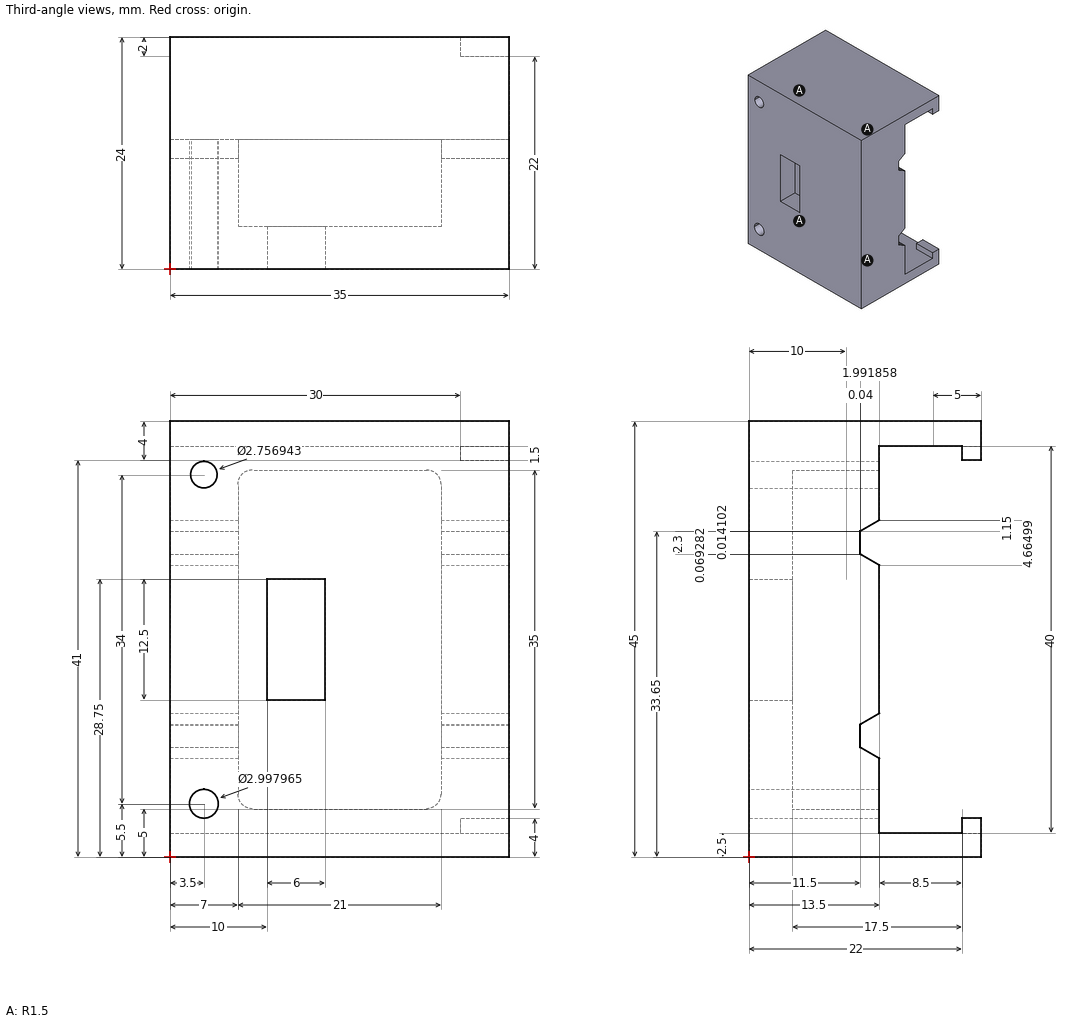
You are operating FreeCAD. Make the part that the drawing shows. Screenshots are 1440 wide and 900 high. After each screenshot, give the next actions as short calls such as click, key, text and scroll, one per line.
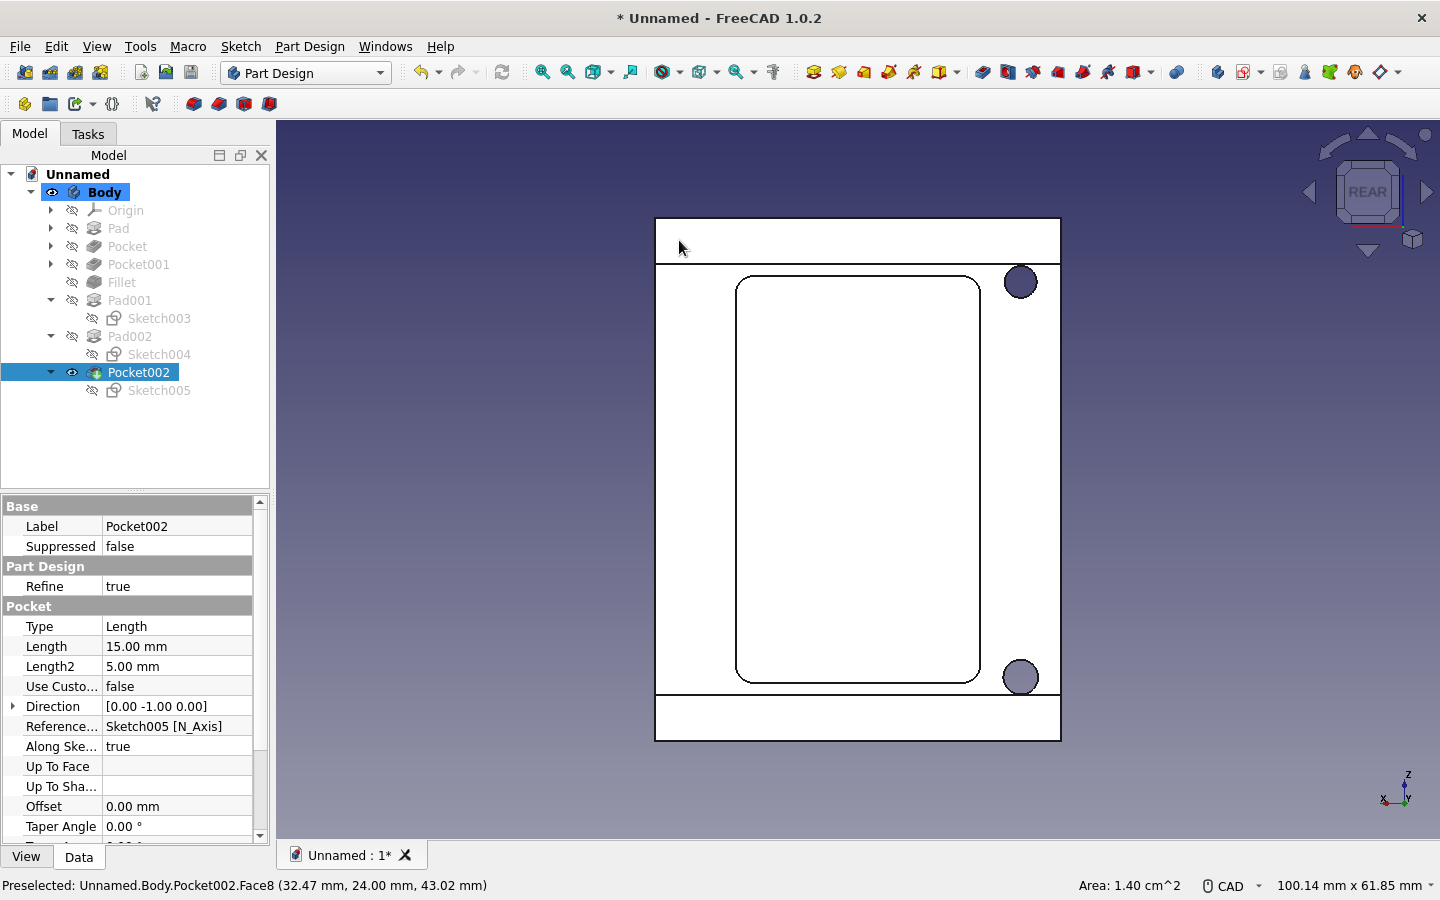
click(1242, 72)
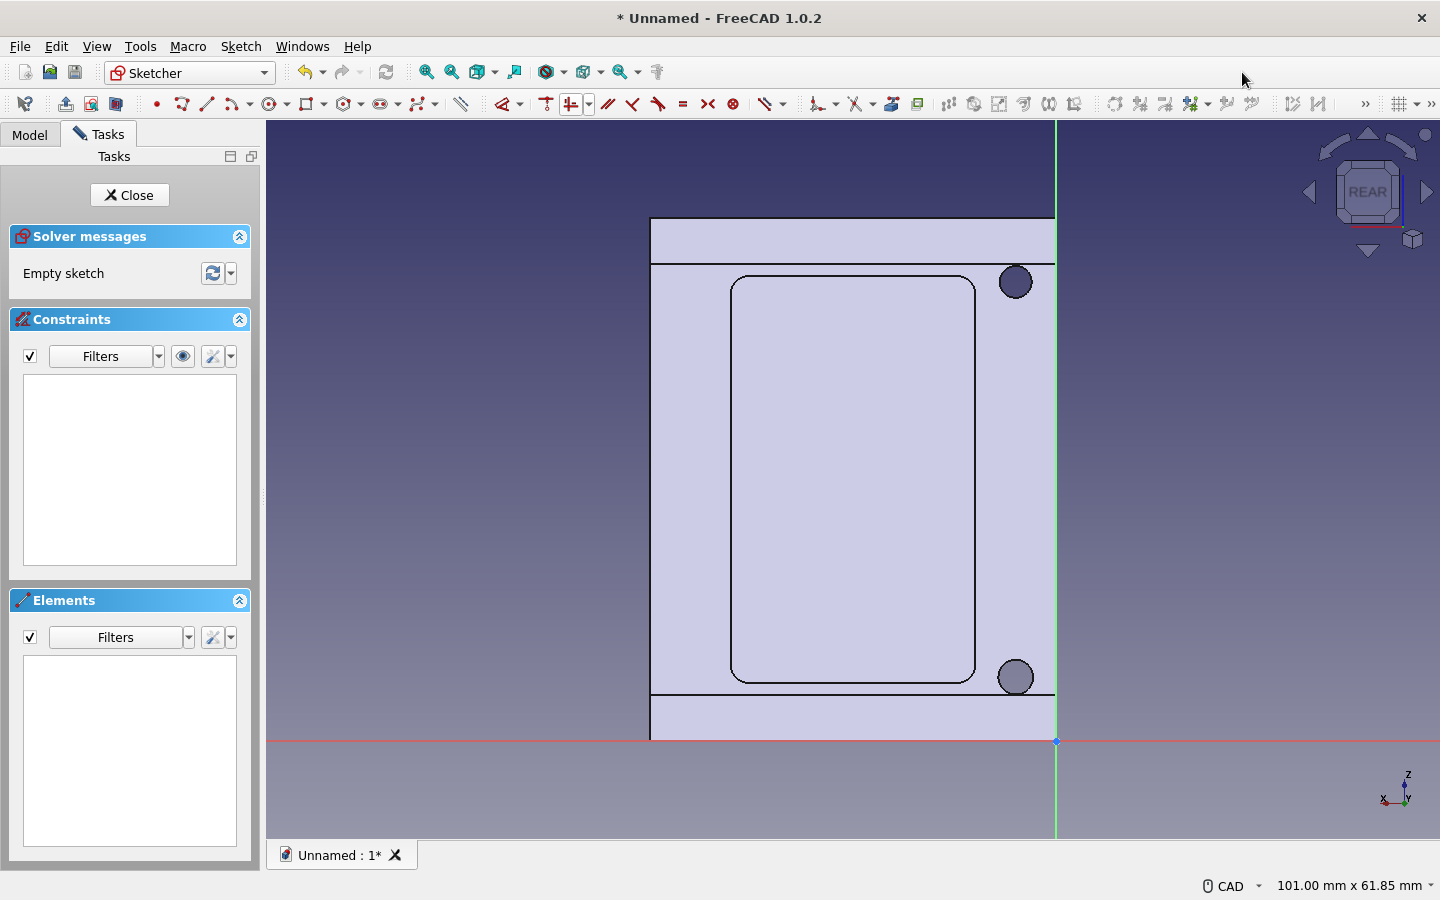
key(g)
key(r)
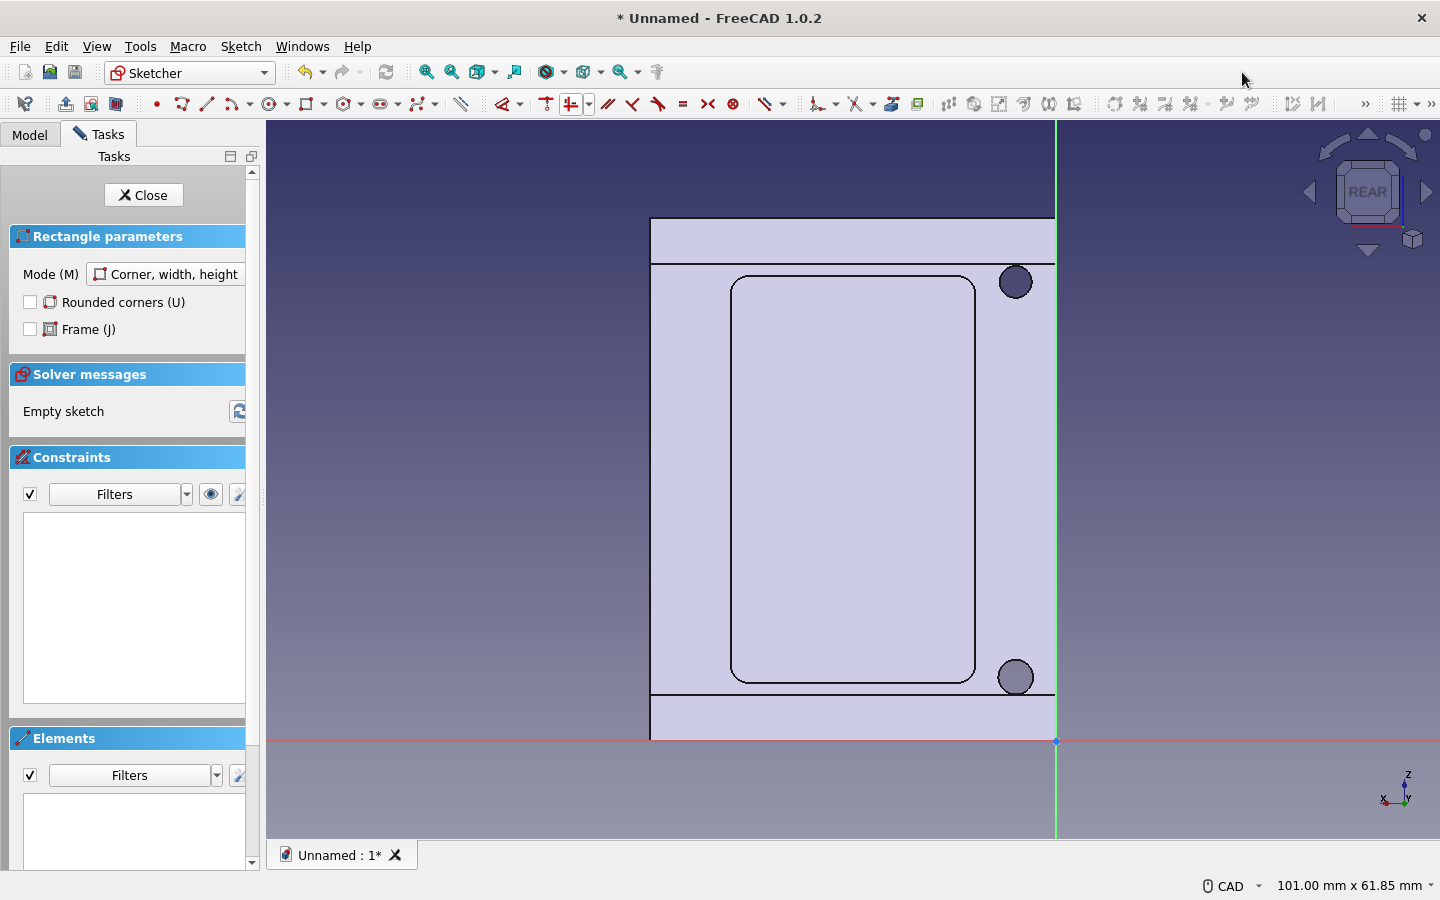
click(708, 247)
click(1056, 264)
key(Escape)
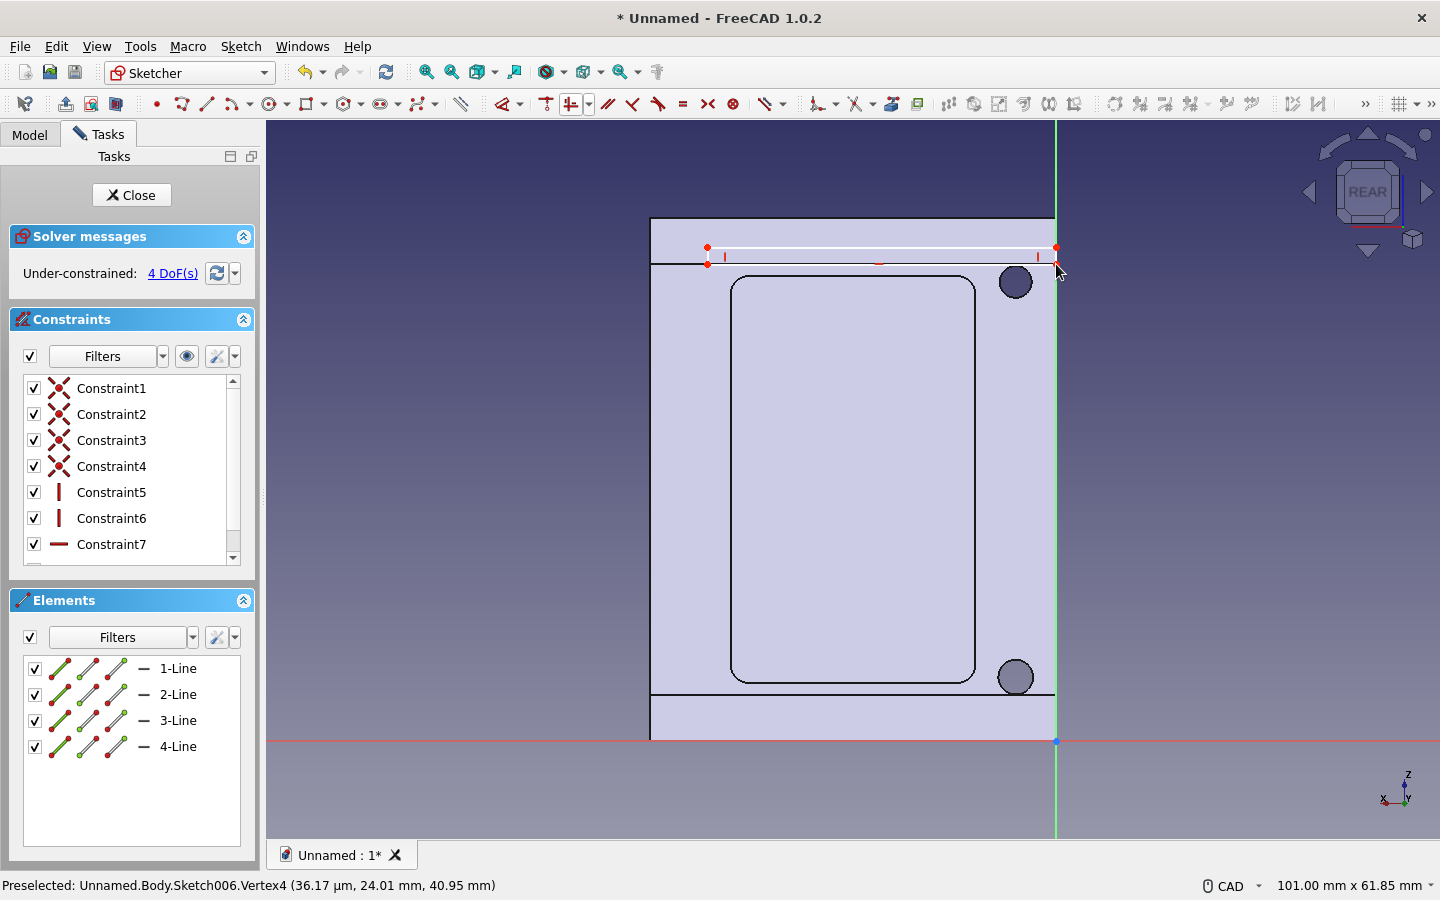
click(1056, 265)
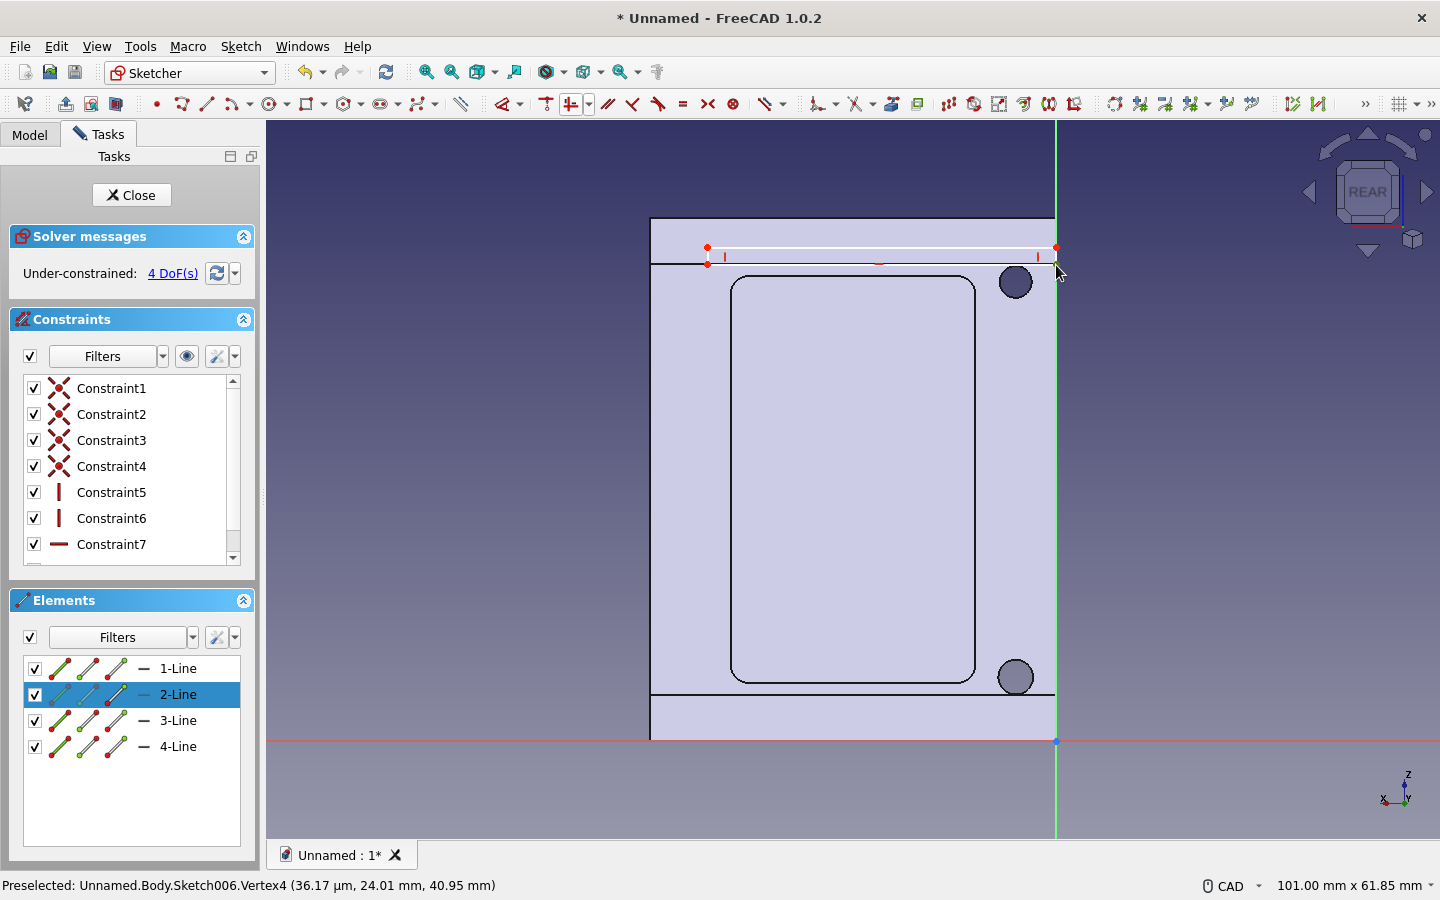
click(1056, 669)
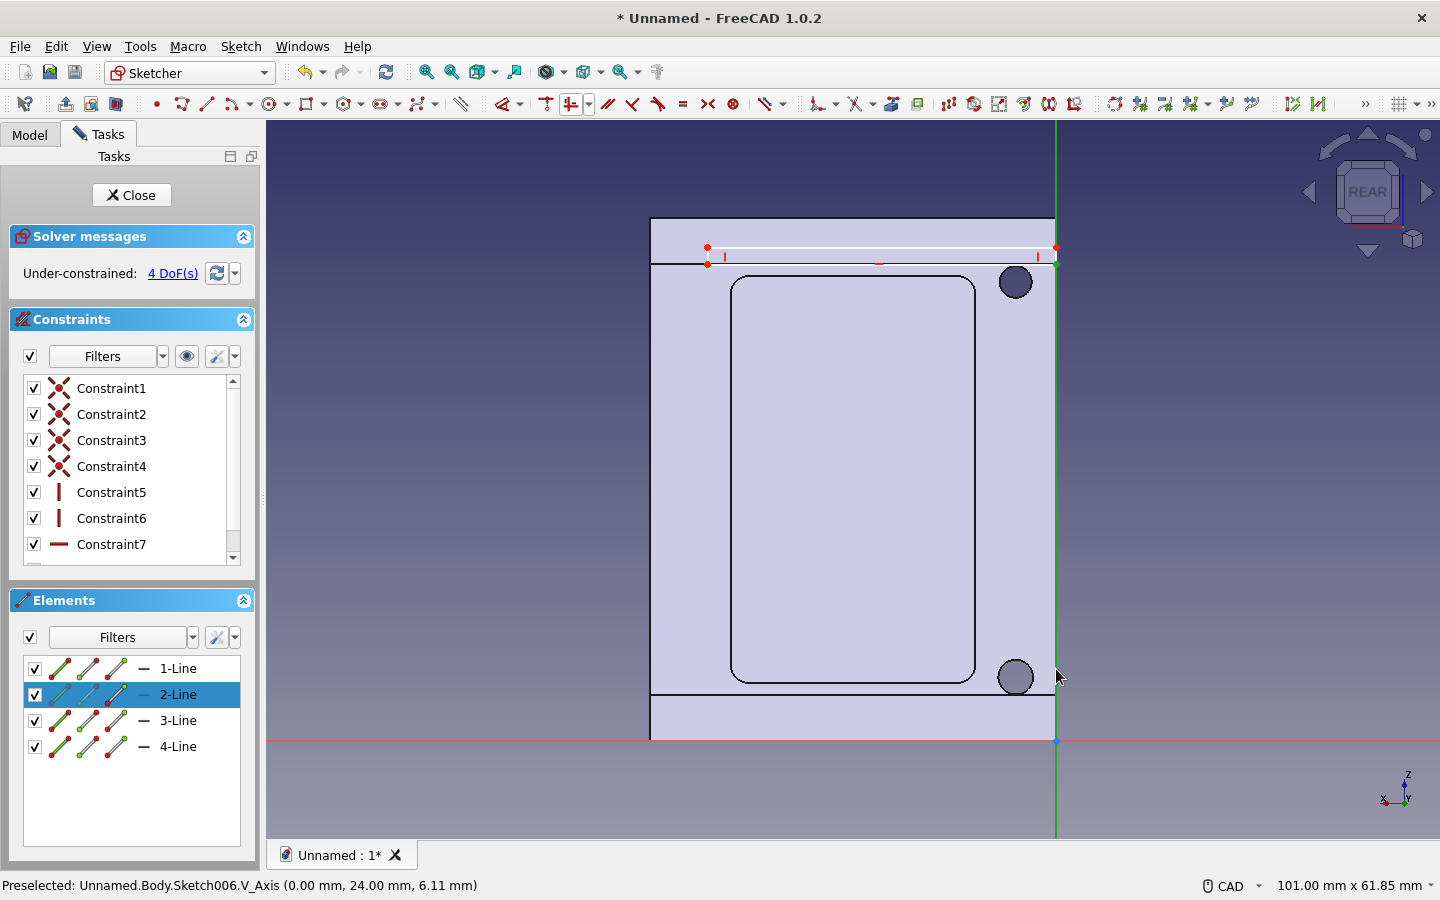
click(546, 104)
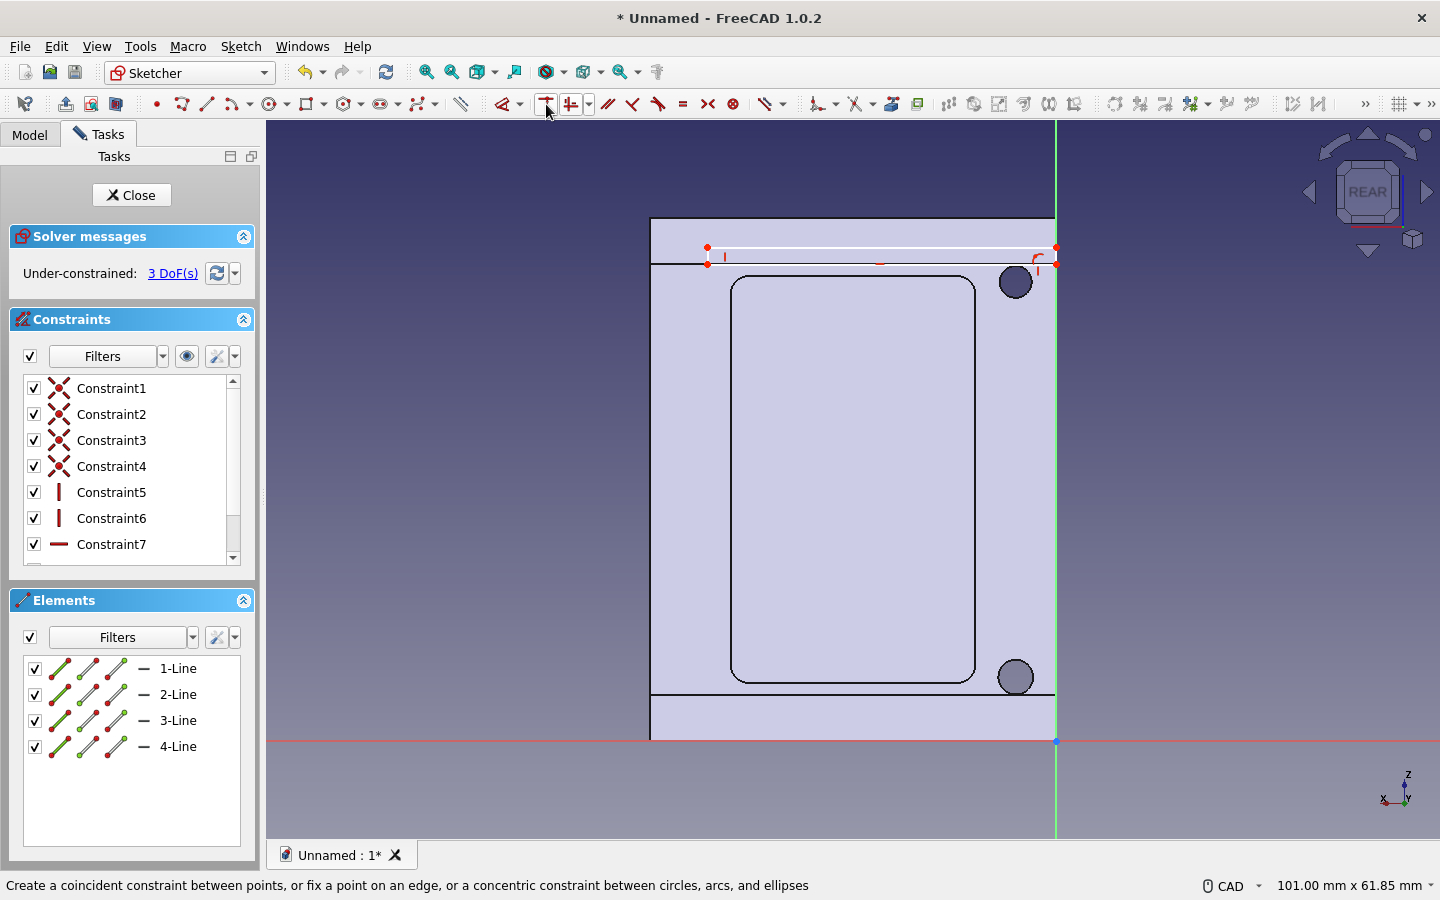
key(d)